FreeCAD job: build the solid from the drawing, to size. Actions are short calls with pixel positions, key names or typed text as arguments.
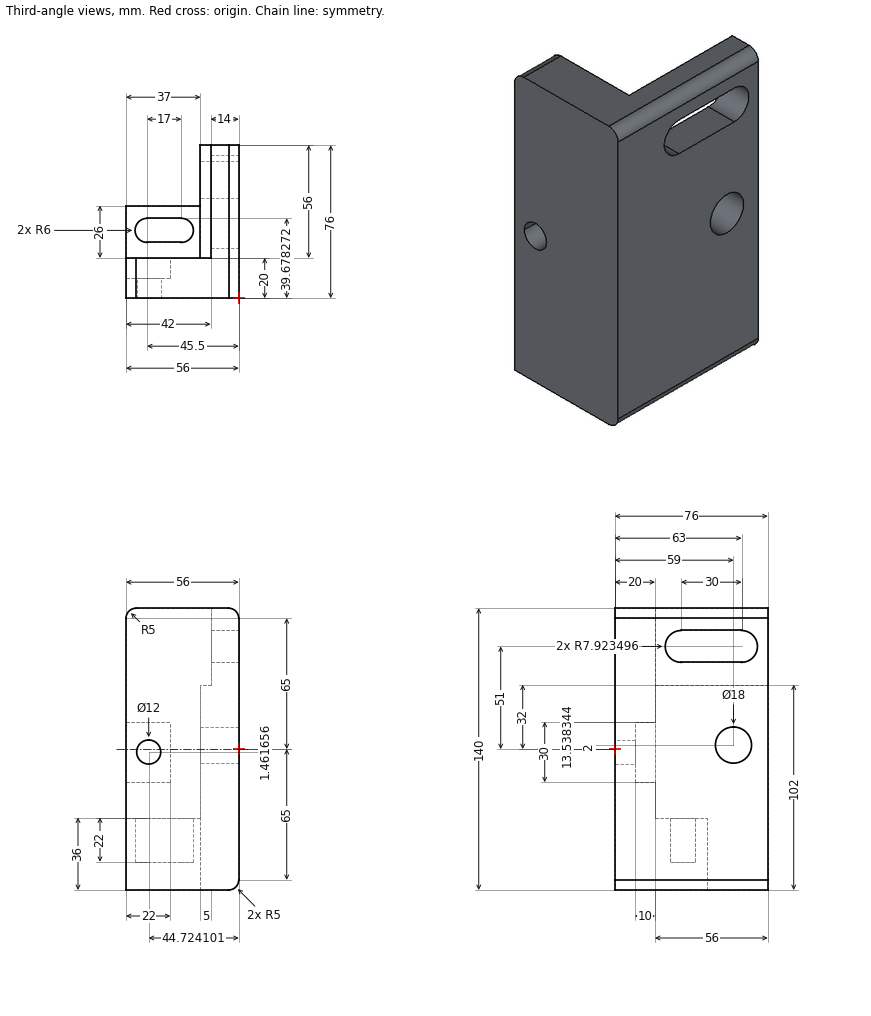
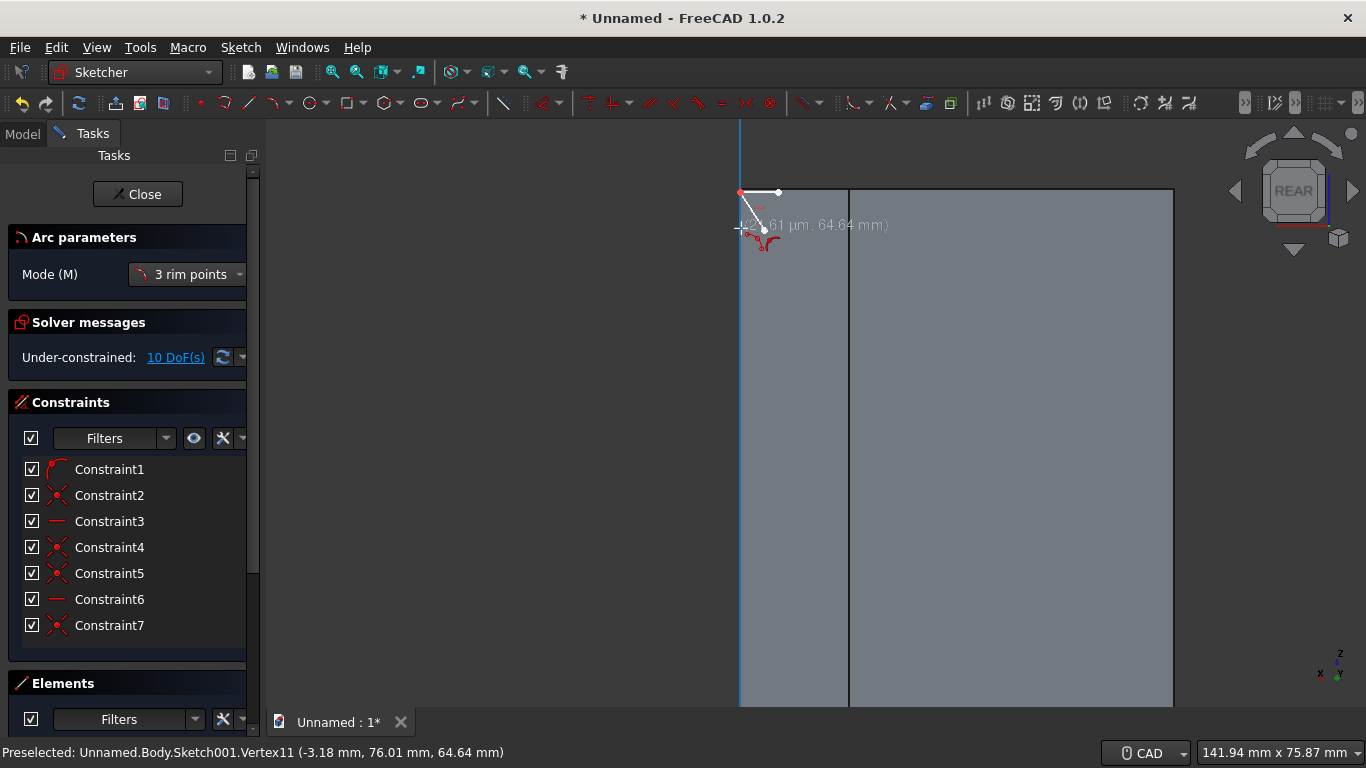
click(765, 230)
click(778, 192)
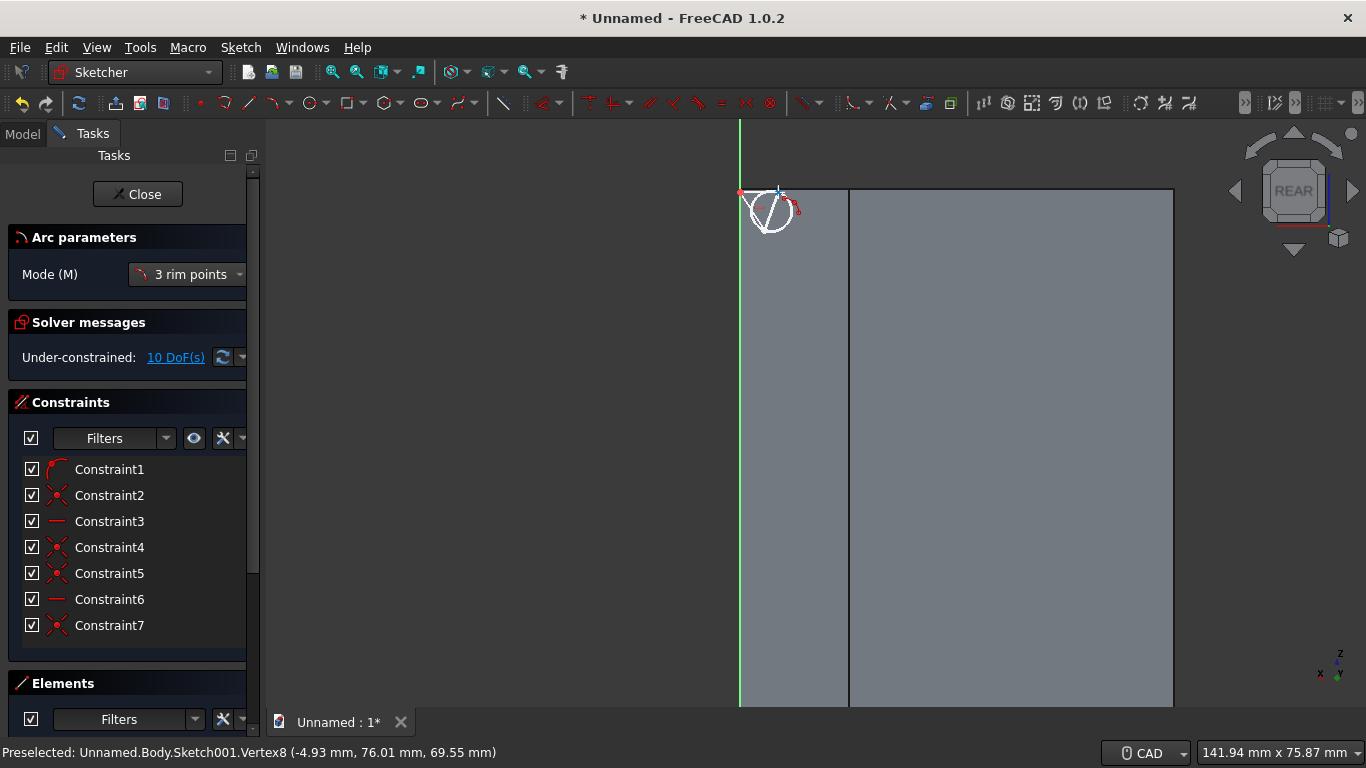
scroll(751, 200, up, 2)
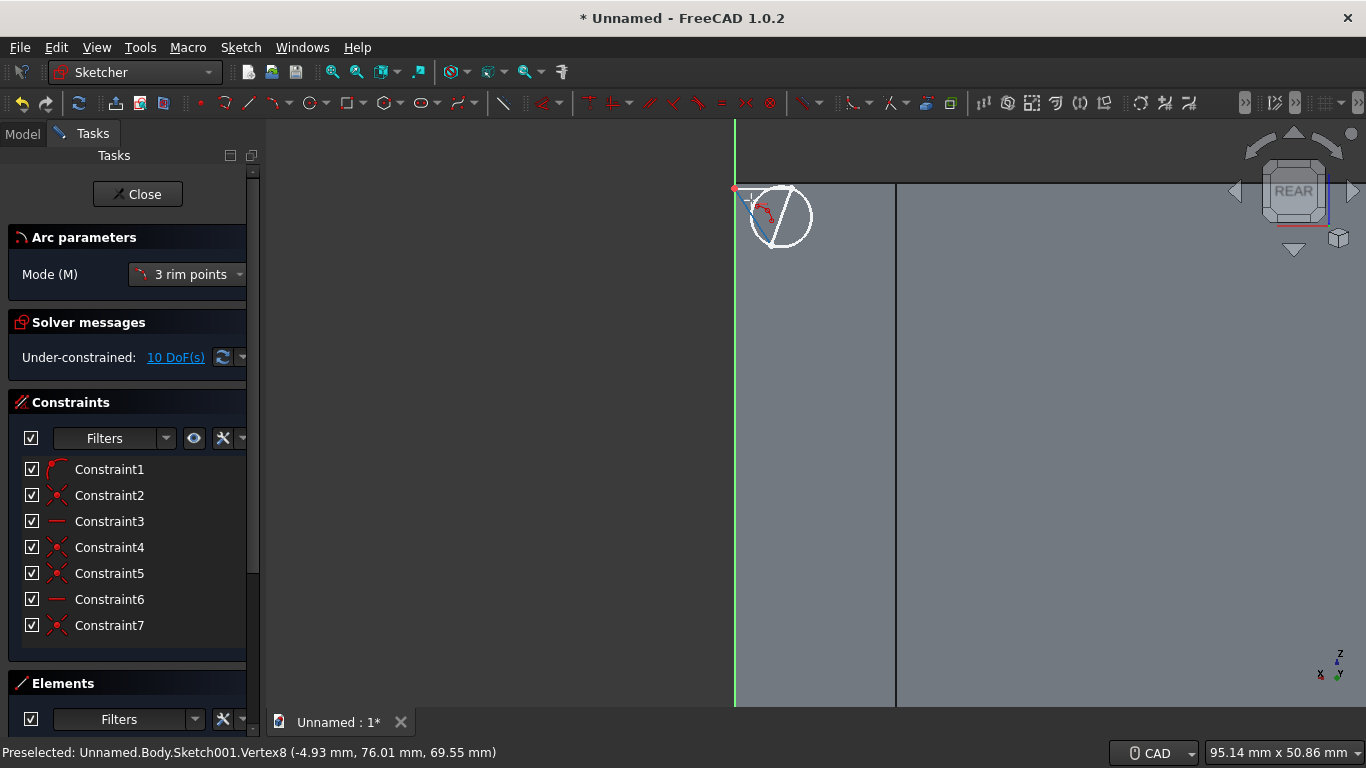
click(751, 200)
key(Escape)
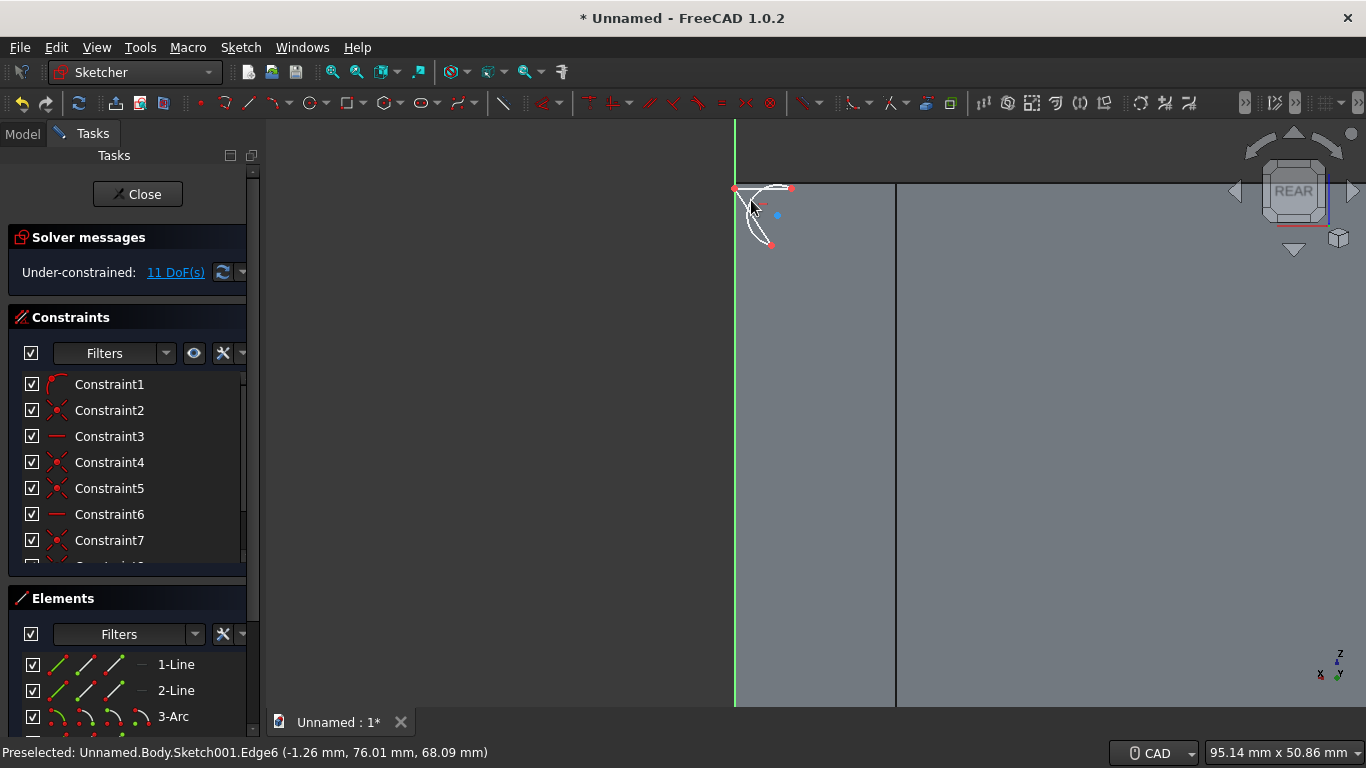
scroll(742, 223, down, 7)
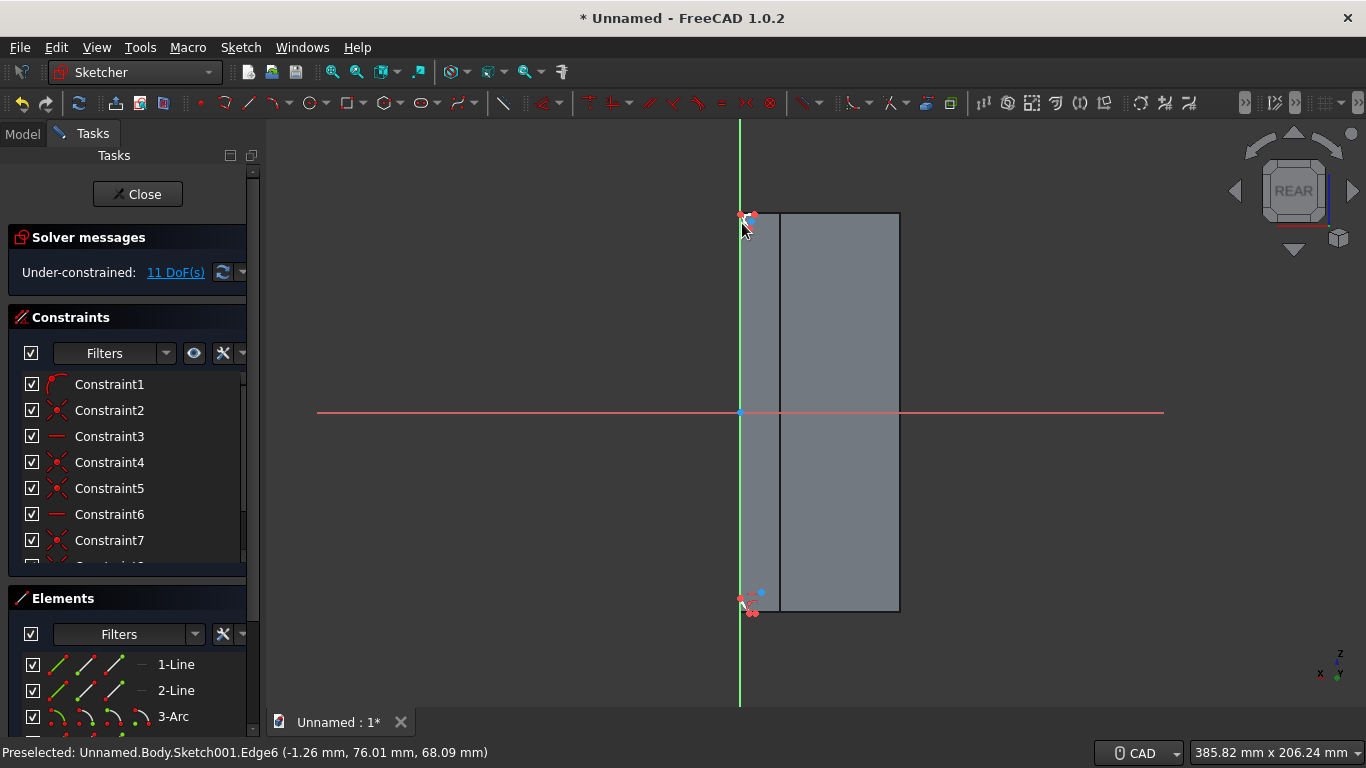
scroll(747, 611, up, 14)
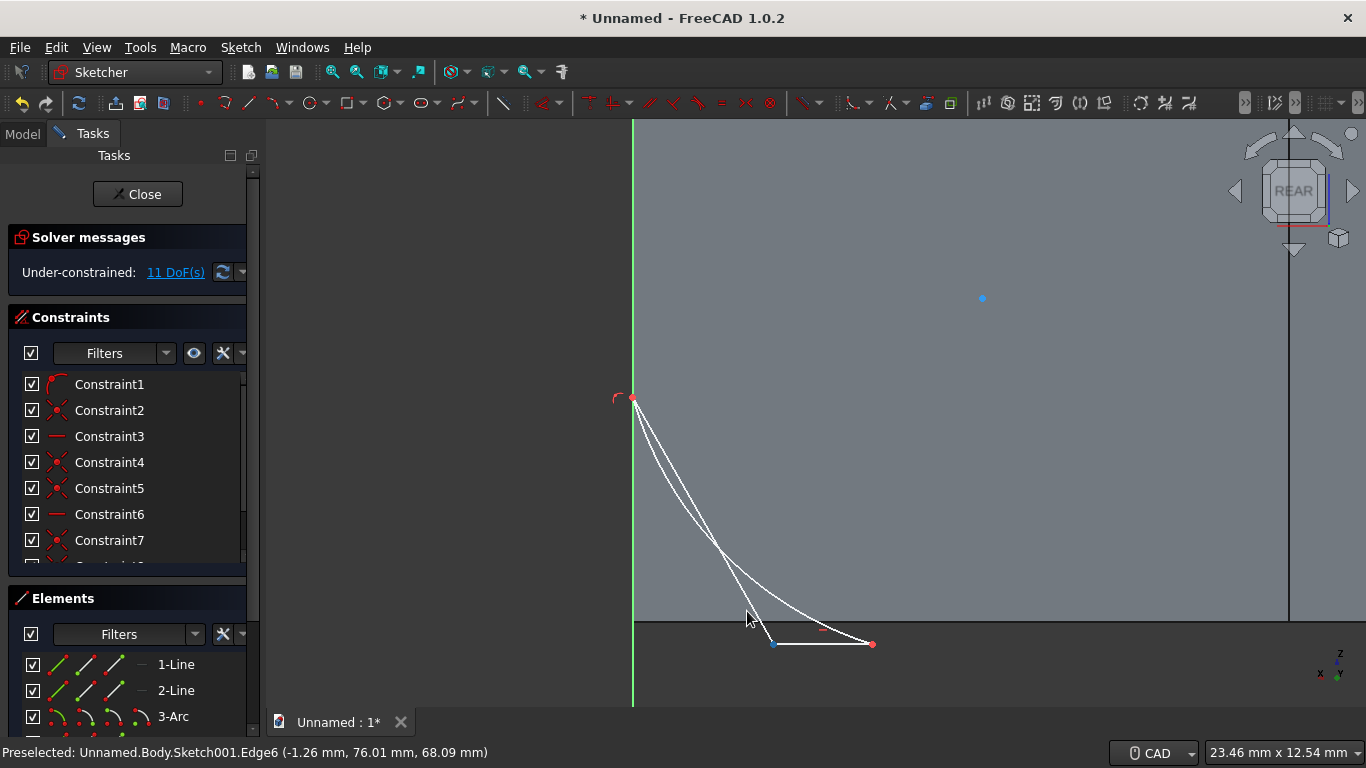
click(746, 595)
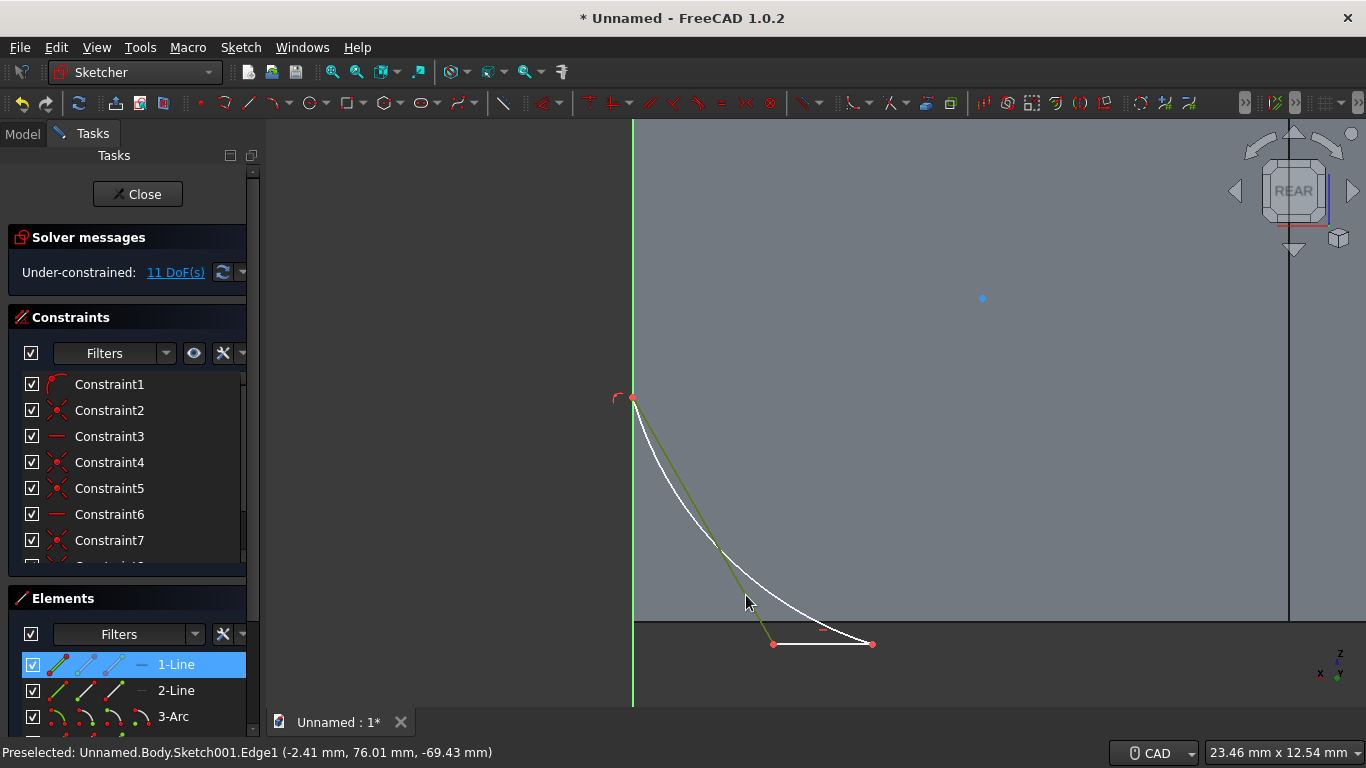
click(677, 495)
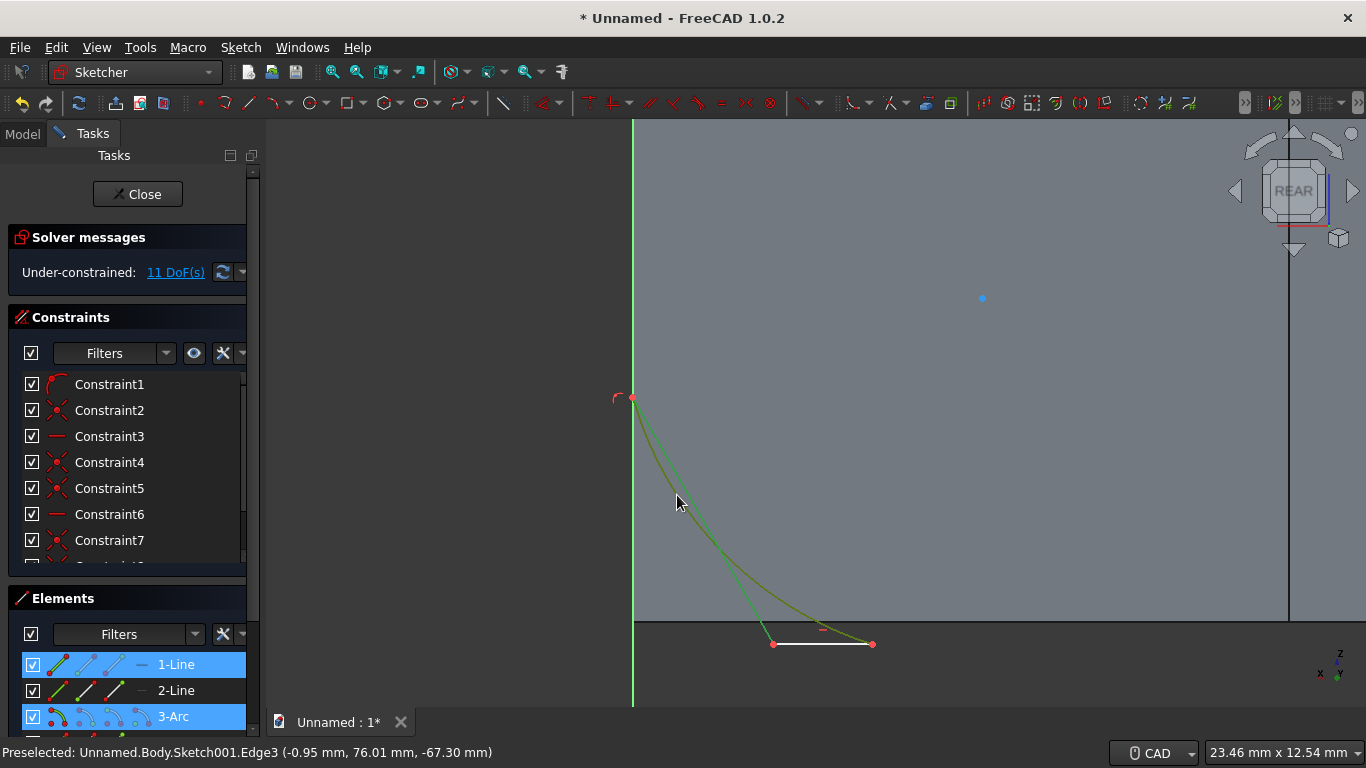
click(698, 104)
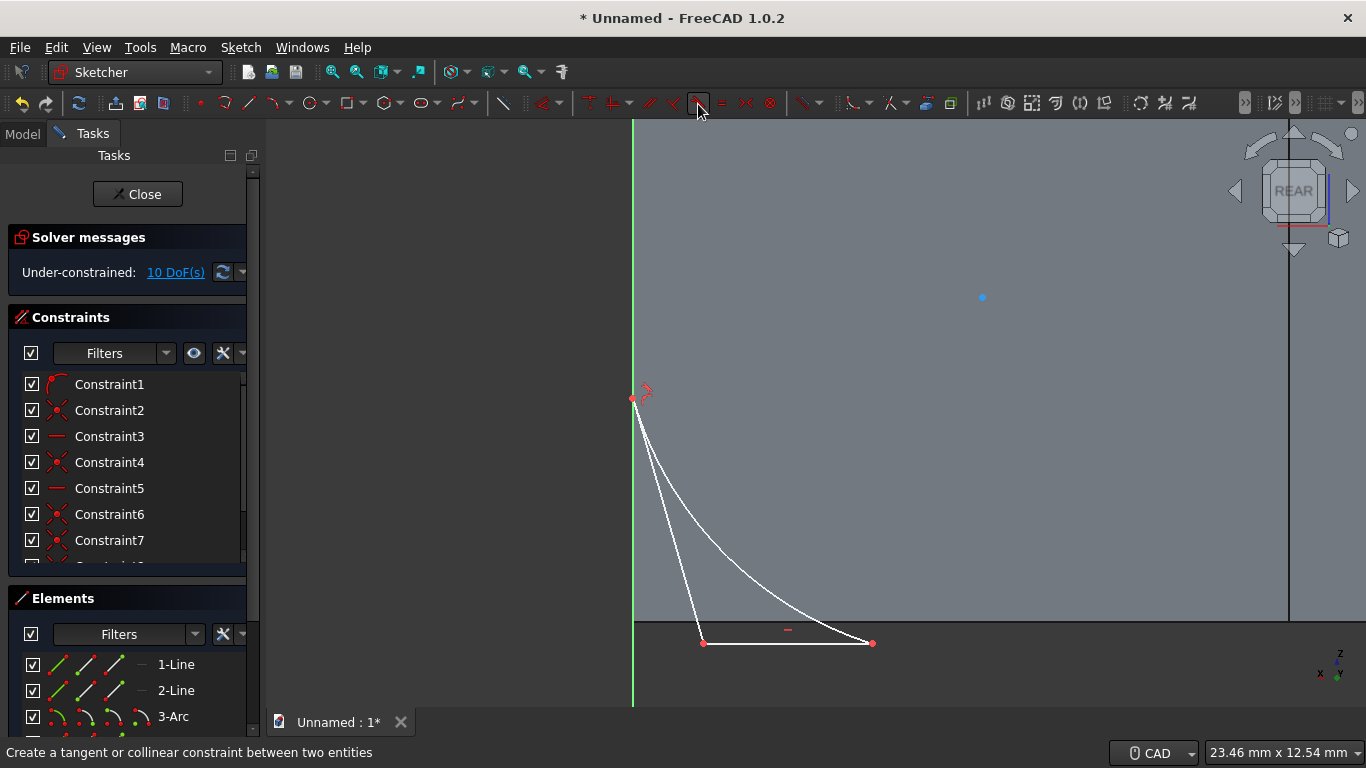
scroll(747, 612, down, 14)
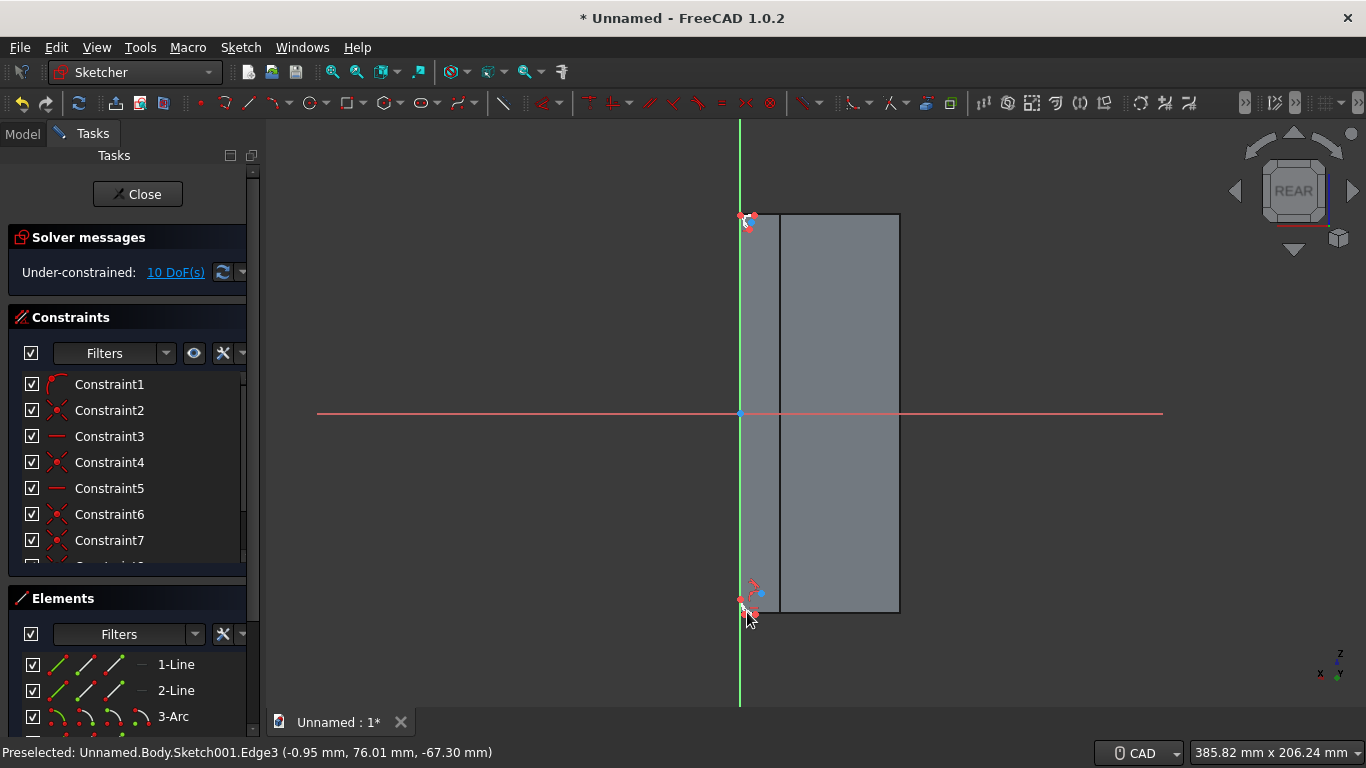
scroll(748, 615, up, 8)